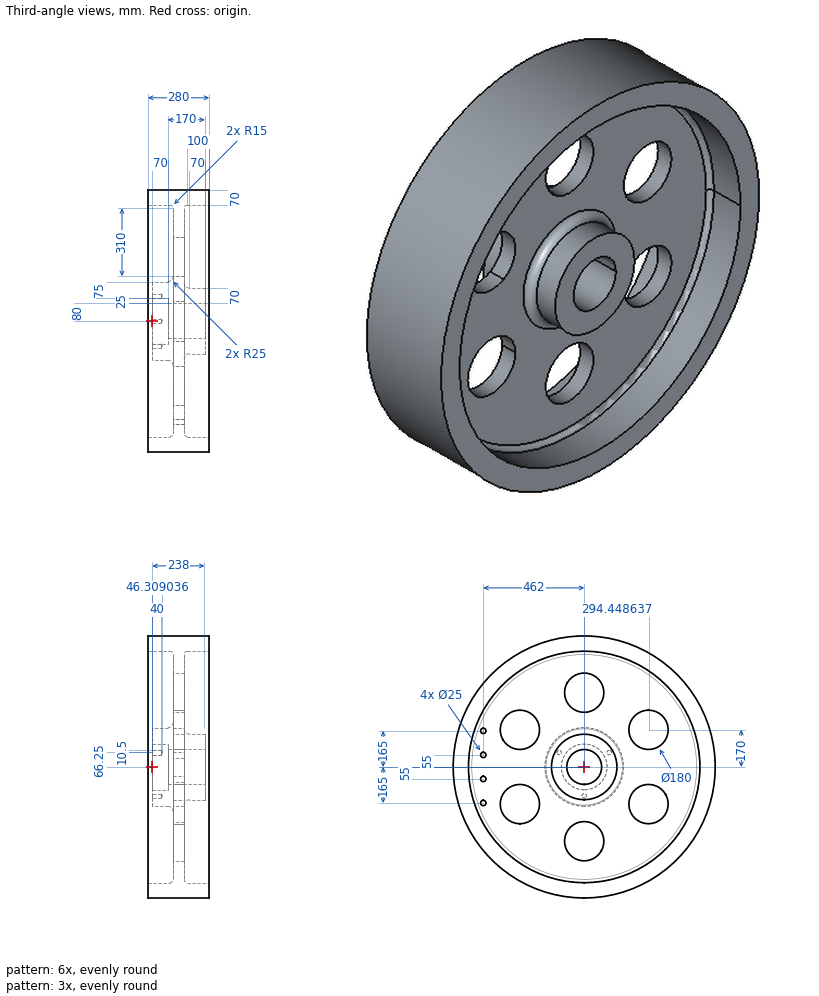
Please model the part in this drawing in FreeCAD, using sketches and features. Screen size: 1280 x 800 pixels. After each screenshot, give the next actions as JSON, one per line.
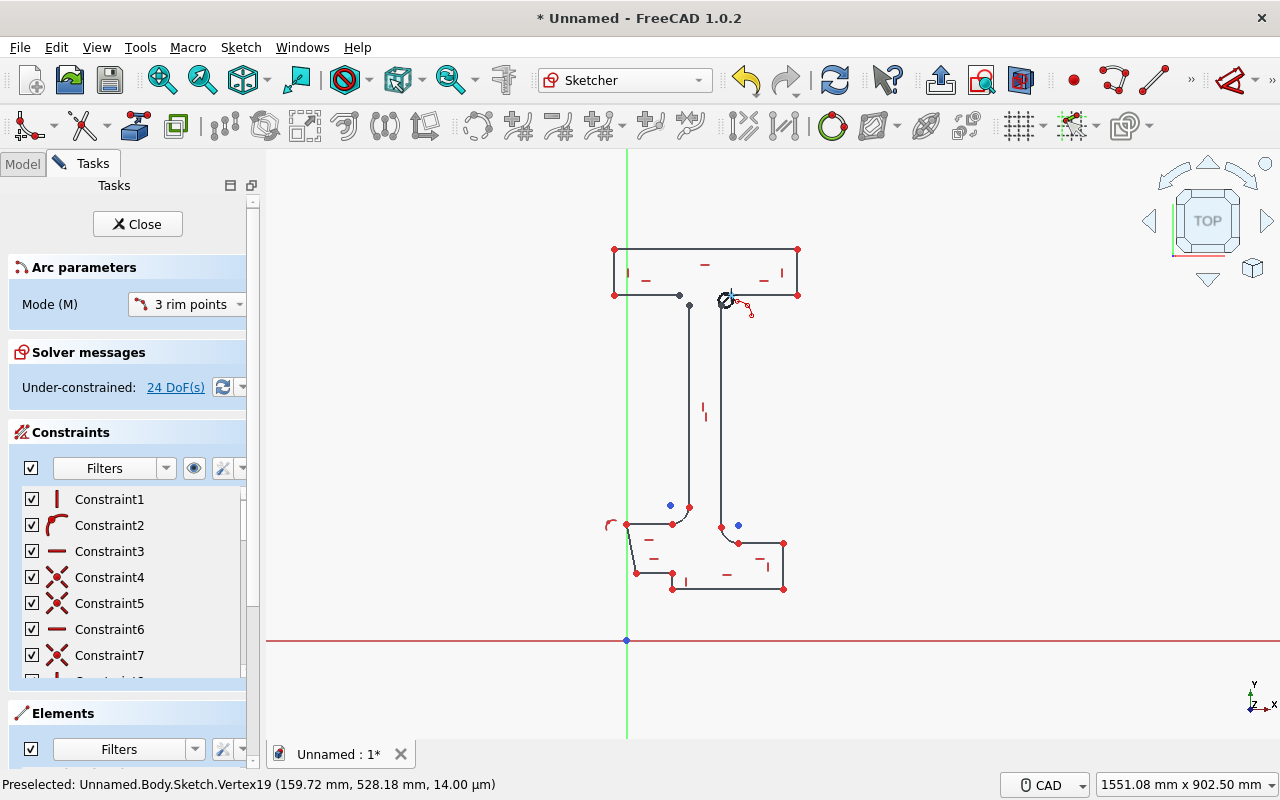
{"action": "scroll", "coordinate": [724, 297], "scroll_direction": "up", "scroll_amount": 9}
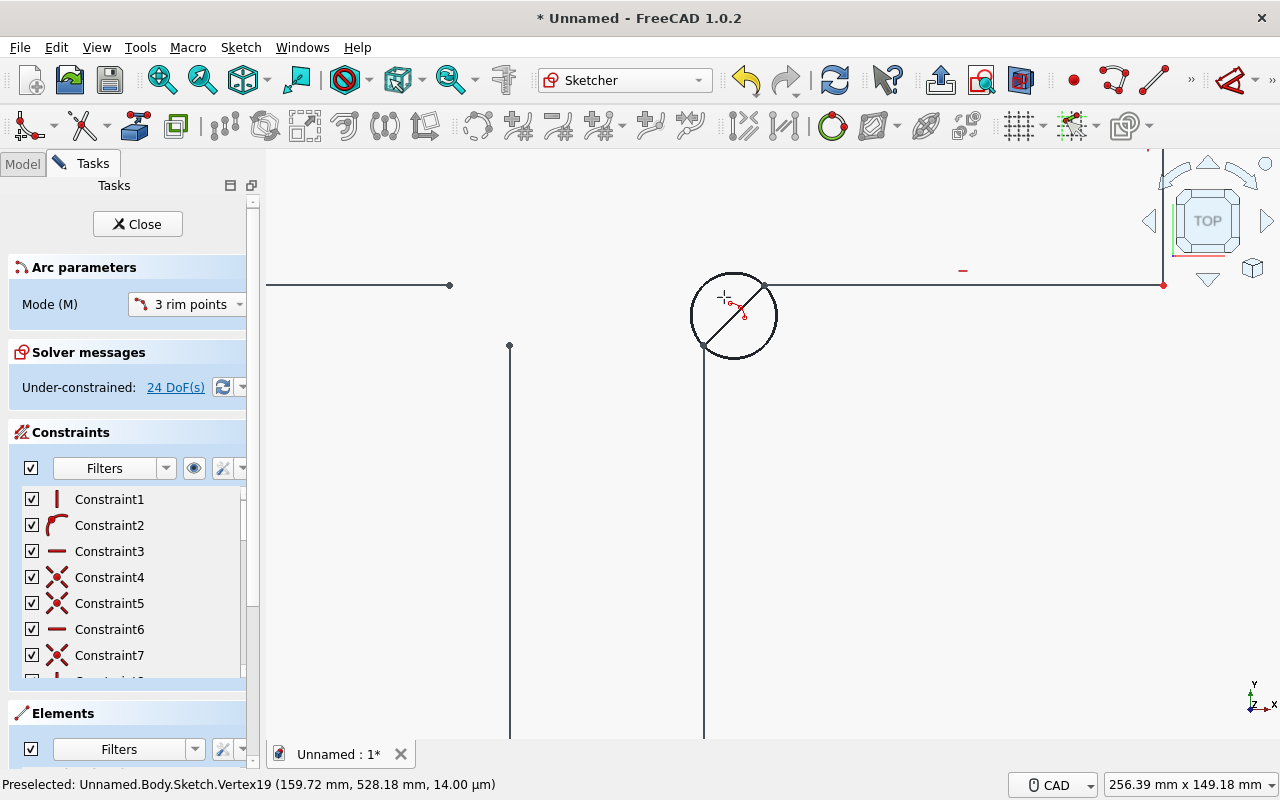
{"action": "left_click", "coordinate": [723, 296]}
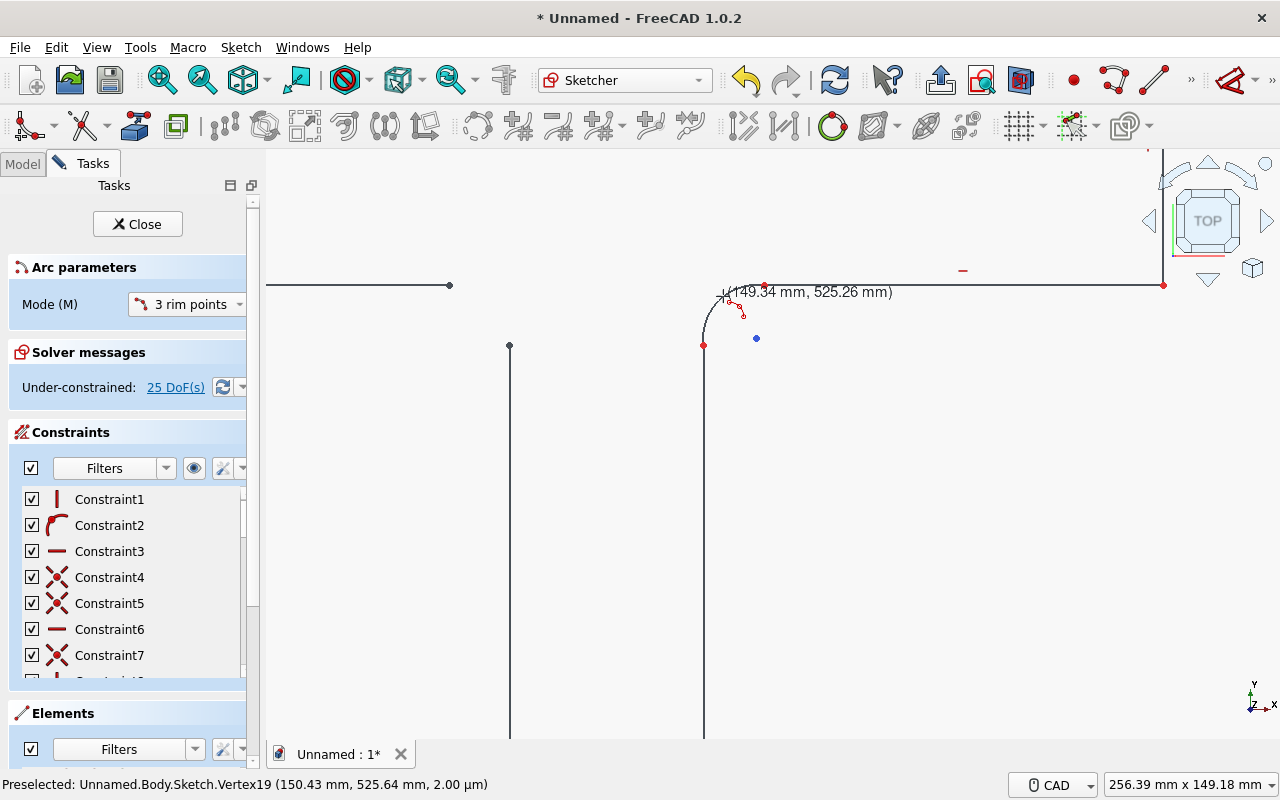
{"action": "scroll", "coordinate": [724, 297], "scroll_direction": "down", "scroll_amount": 9}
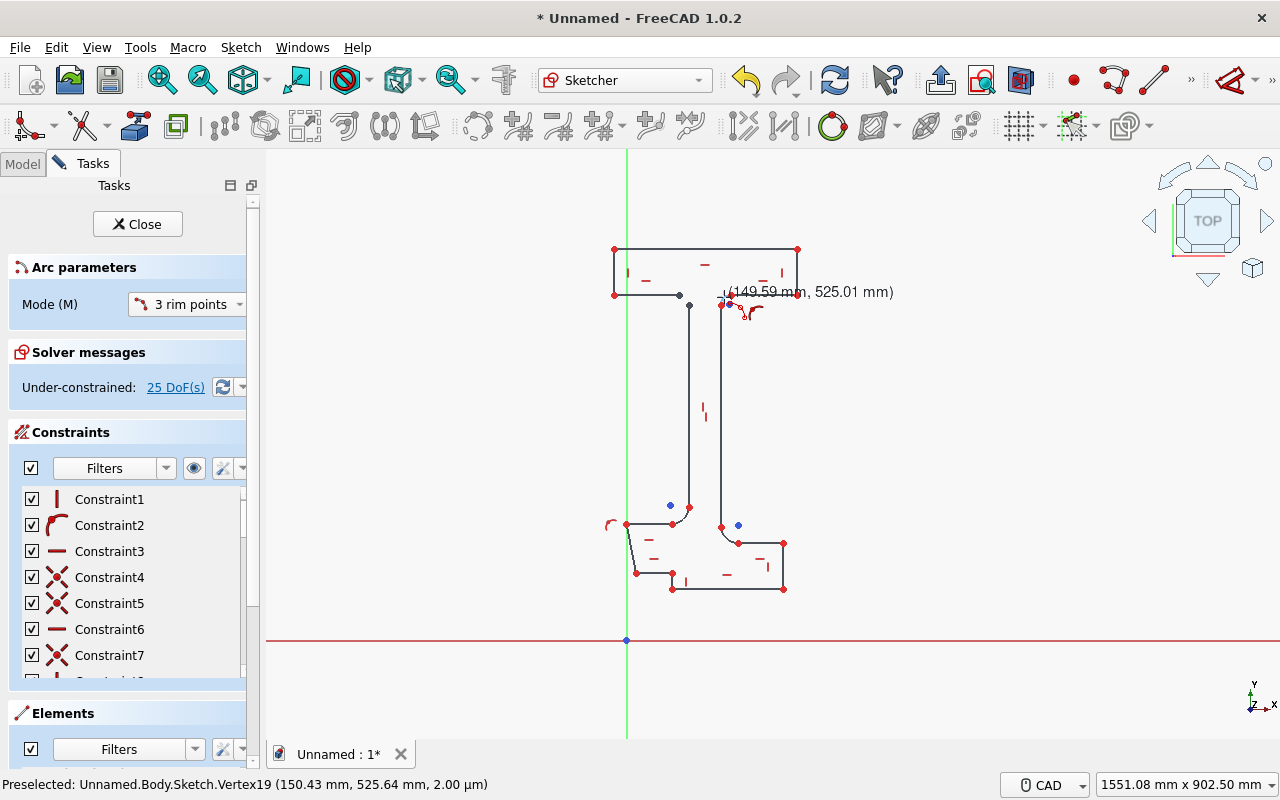
{"action": "left_click", "coordinate": [679, 295]}
{"action": "left_click", "coordinate": [689, 305]}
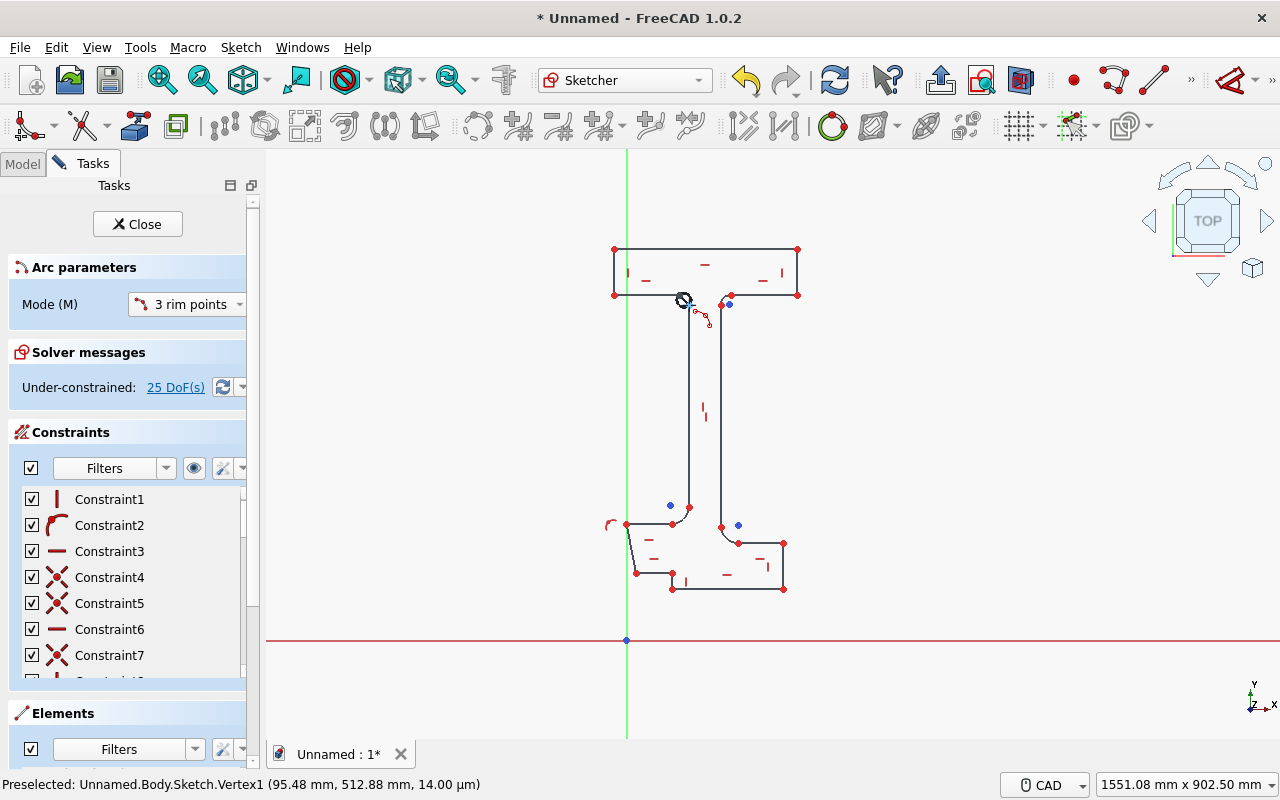
{"action": "scroll", "coordinate": [686, 297], "scroll_direction": "up", "scroll_amount": 9}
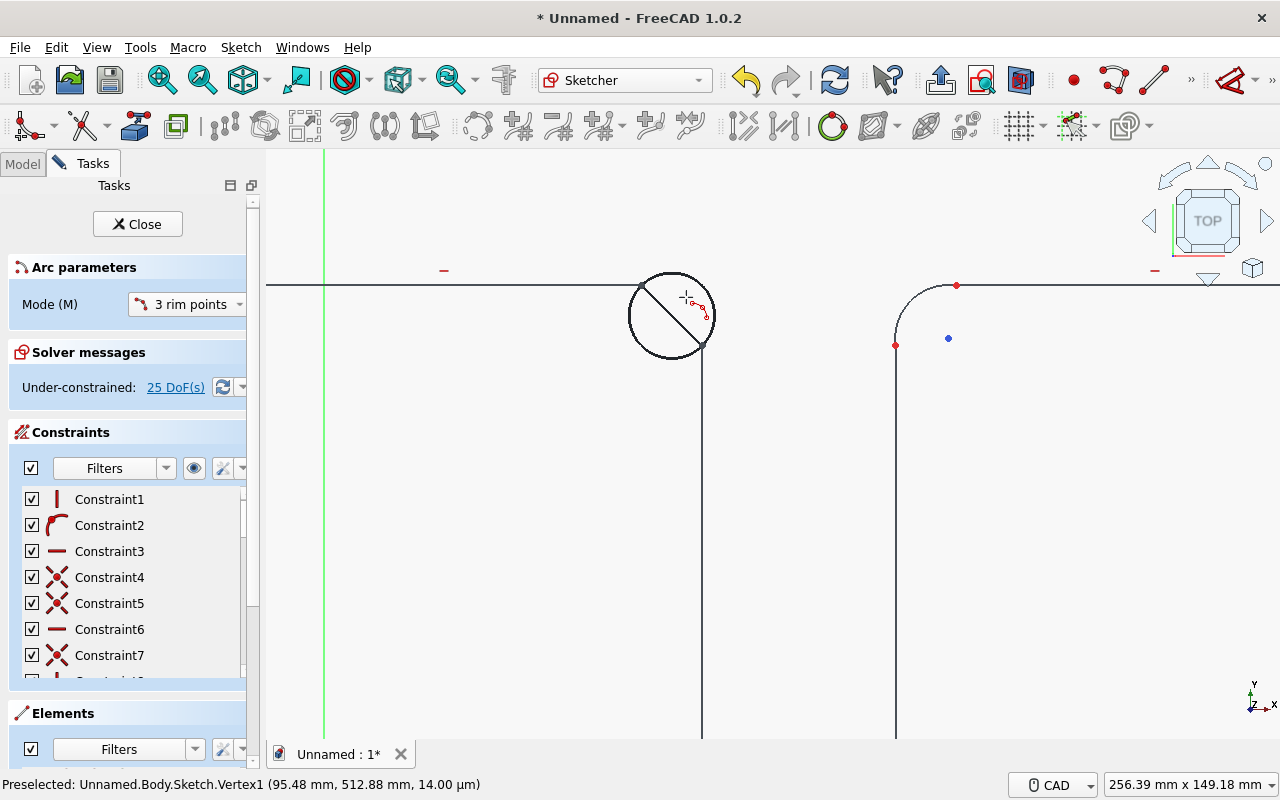
{"action": "left_click", "coordinate": [683, 296]}
{"action": "key", "text": "Escape"}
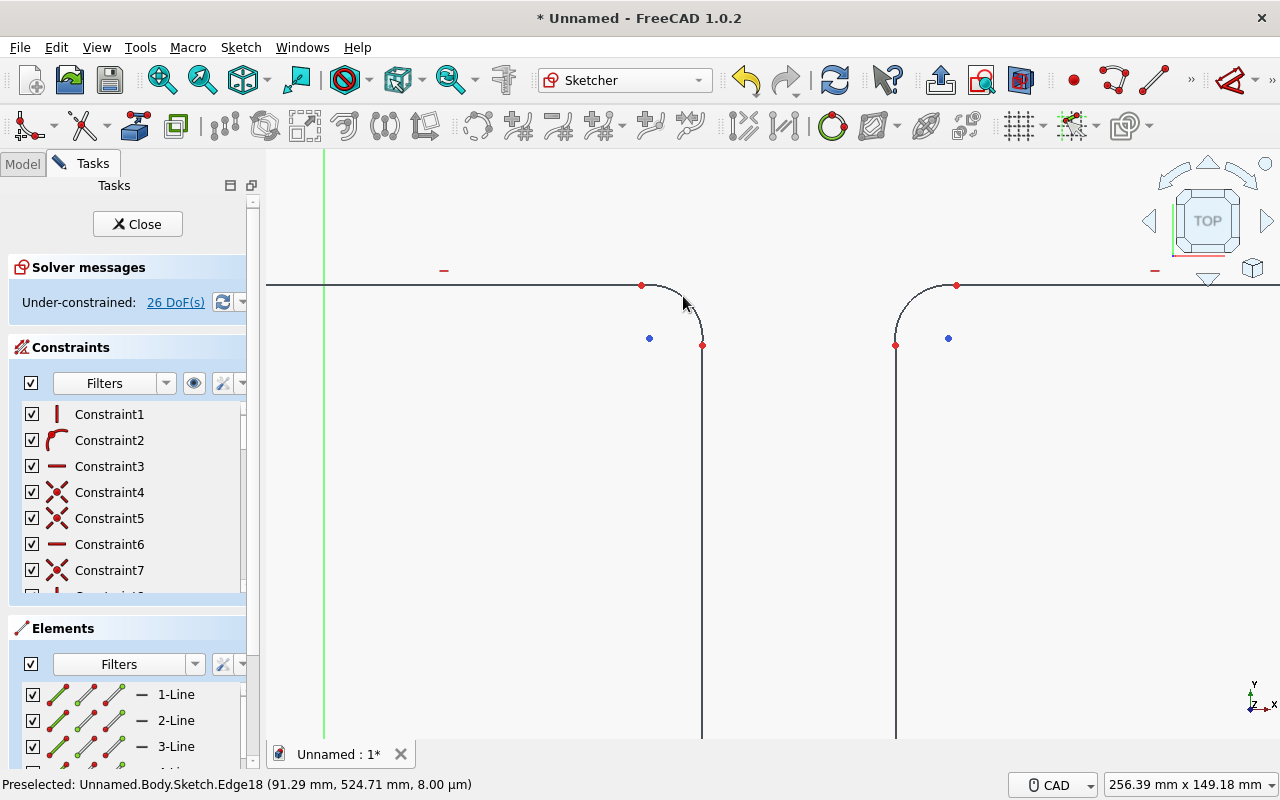
{"action": "scroll", "coordinate": [686, 297], "scroll_direction": "down", "scroll_amount": 9}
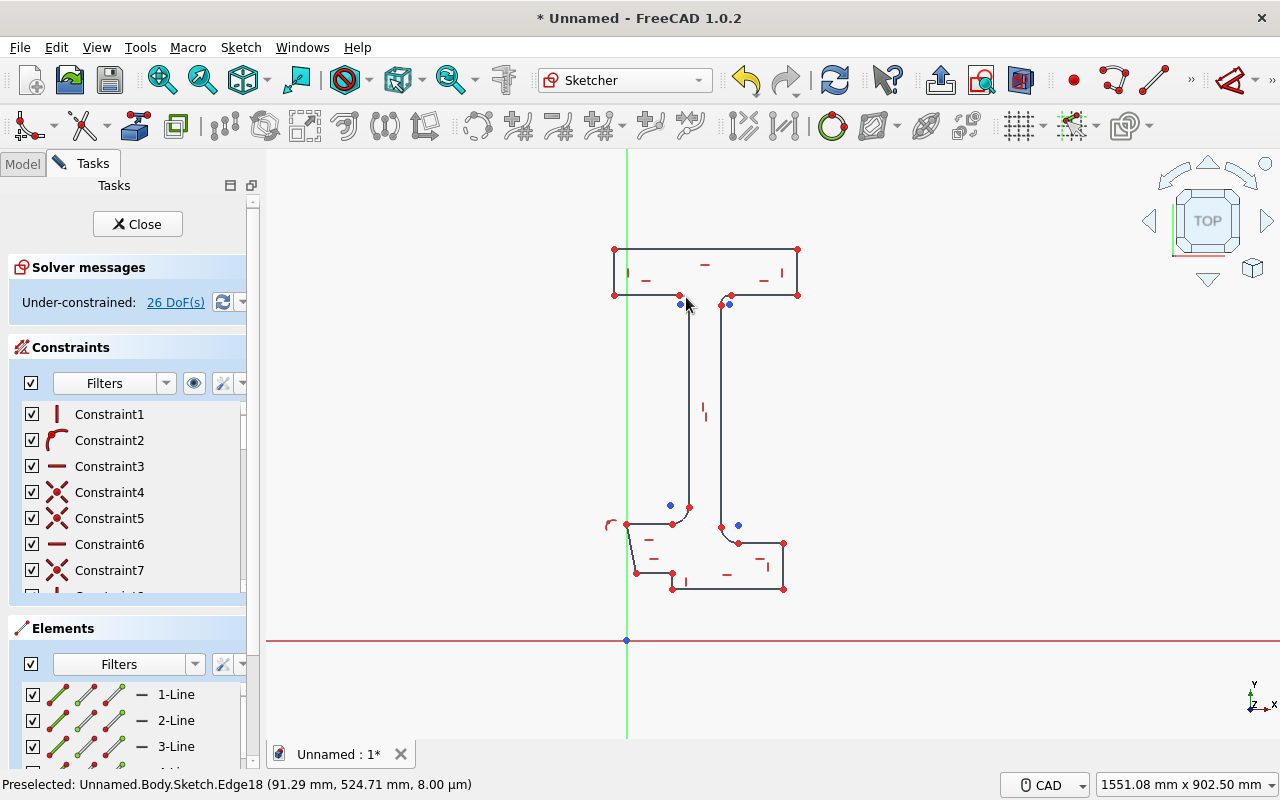
{"action": "left_click", "coordinate": [689, 346]}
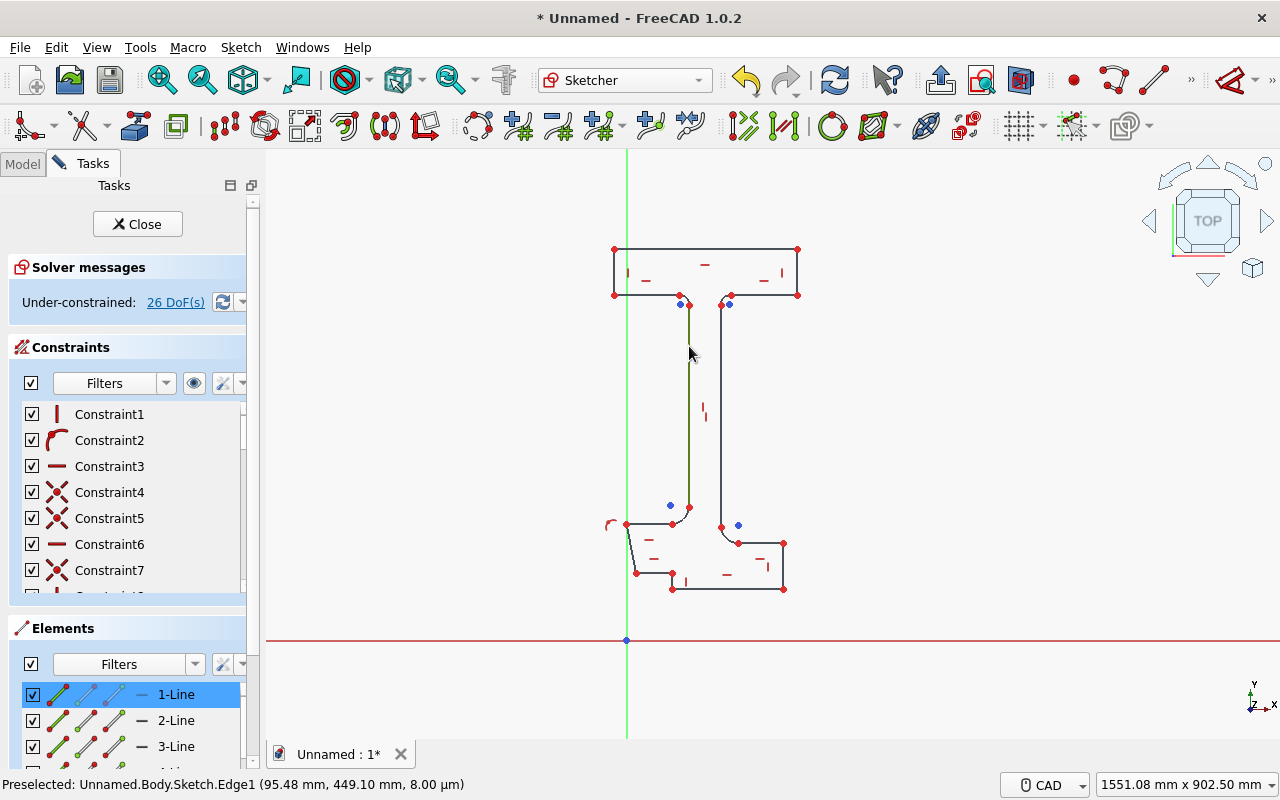
{"action": "left_click", "coordinate": [684, 519]}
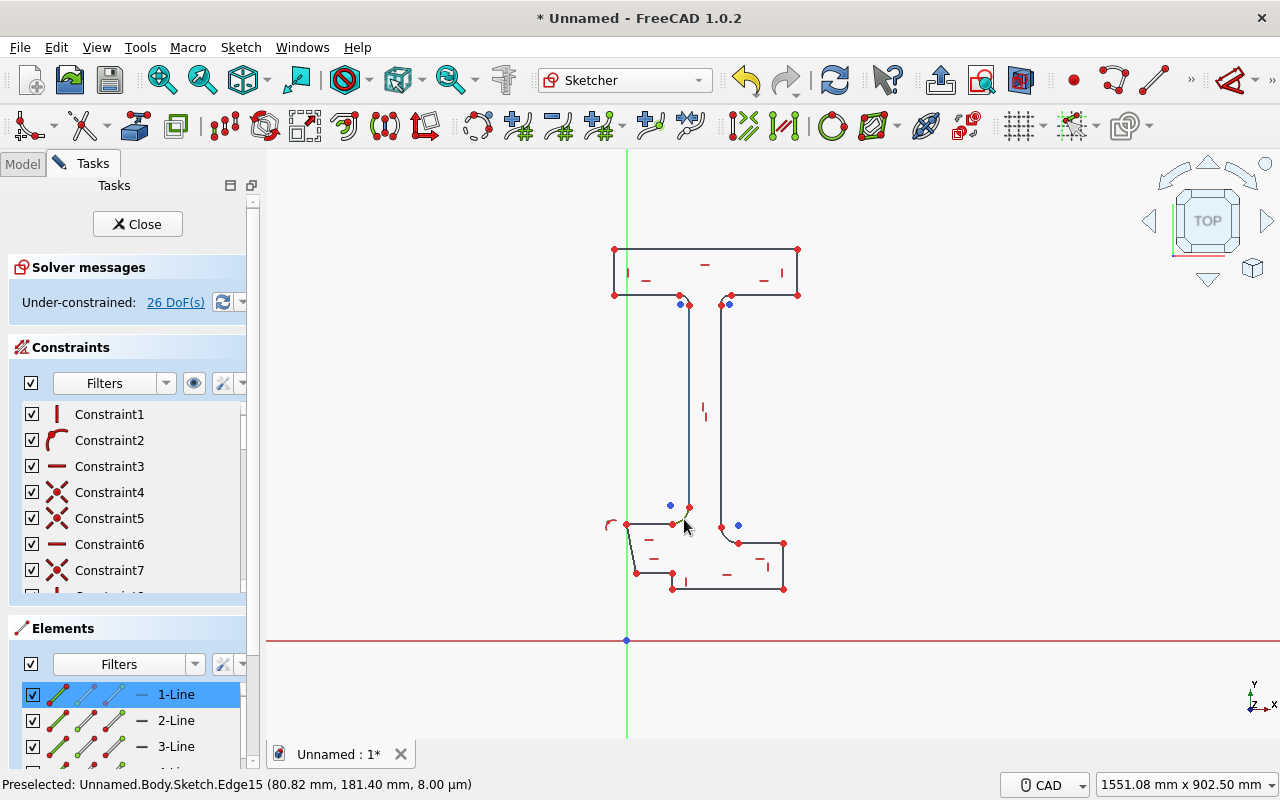
{"action": "key", "text": "t"}